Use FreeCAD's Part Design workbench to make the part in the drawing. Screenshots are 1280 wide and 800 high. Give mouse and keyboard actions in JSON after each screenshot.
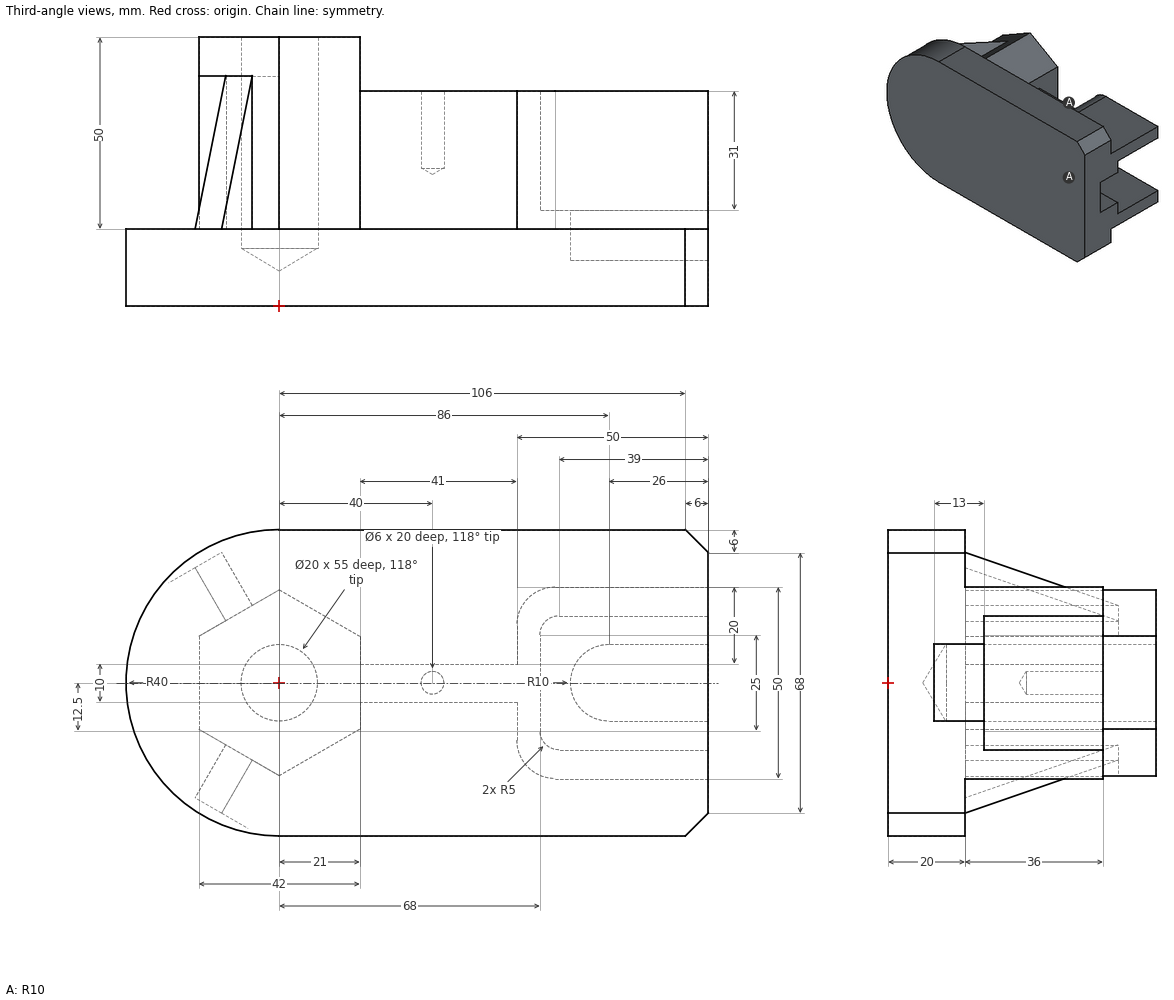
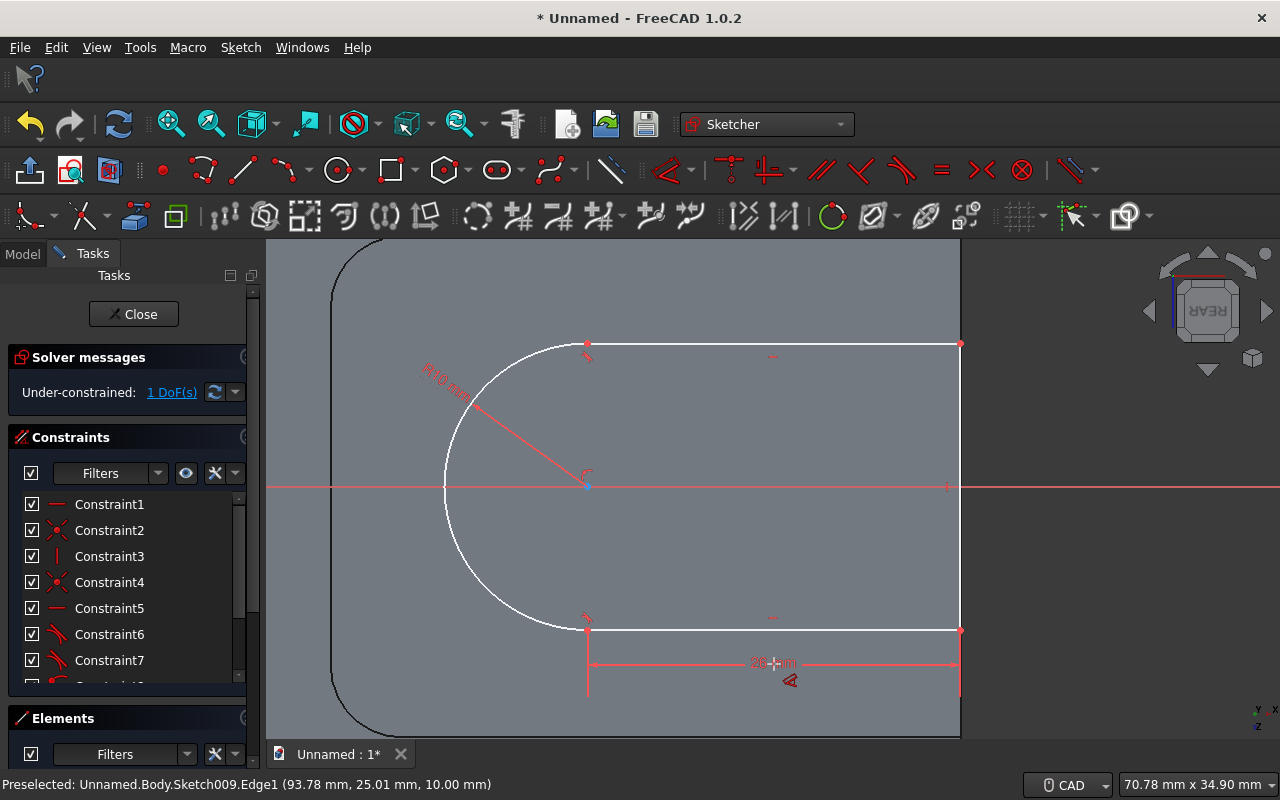
{"action": "left_click", "coordinate": [588, 630]}
{"action": "left_click", "coordinate": [441, 664]}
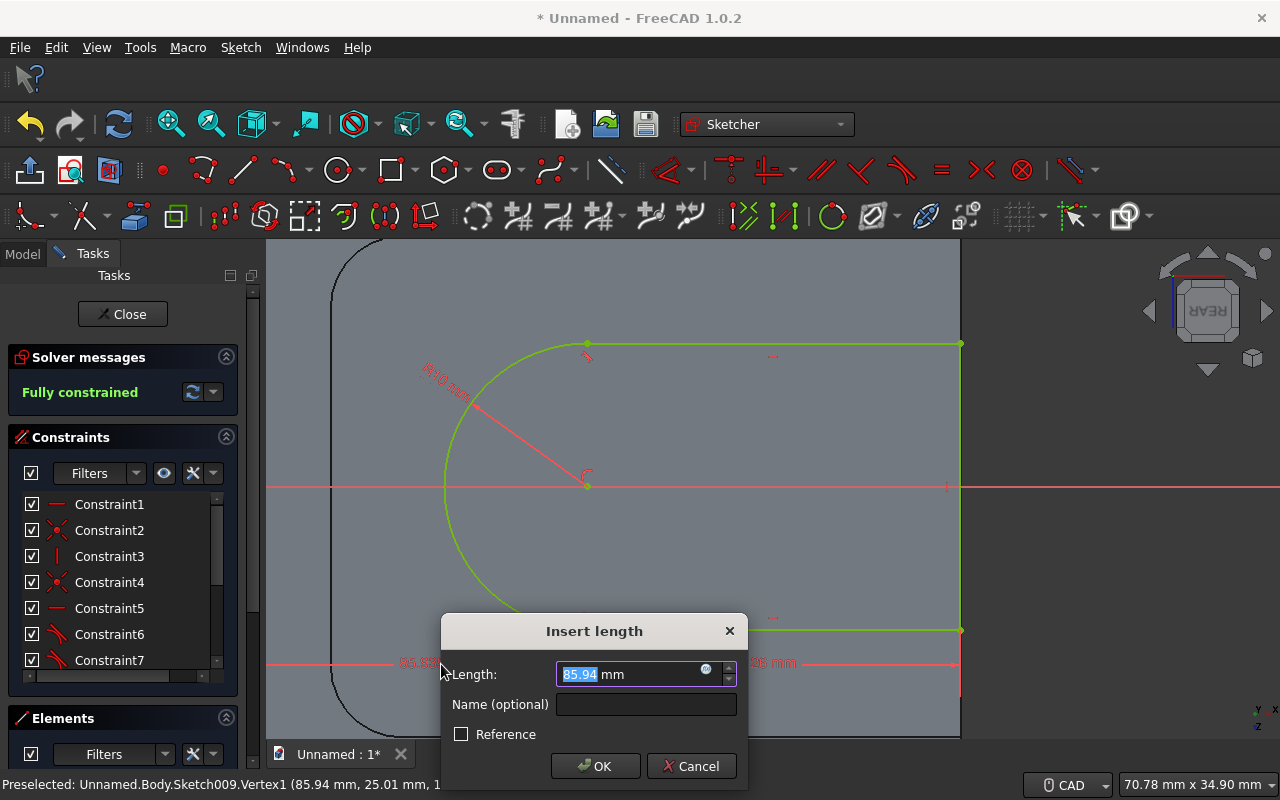
{"action": "type", "text": "86"}
{"action": "key", "text": "Return"}
{"action": "key", "text": "Escape"}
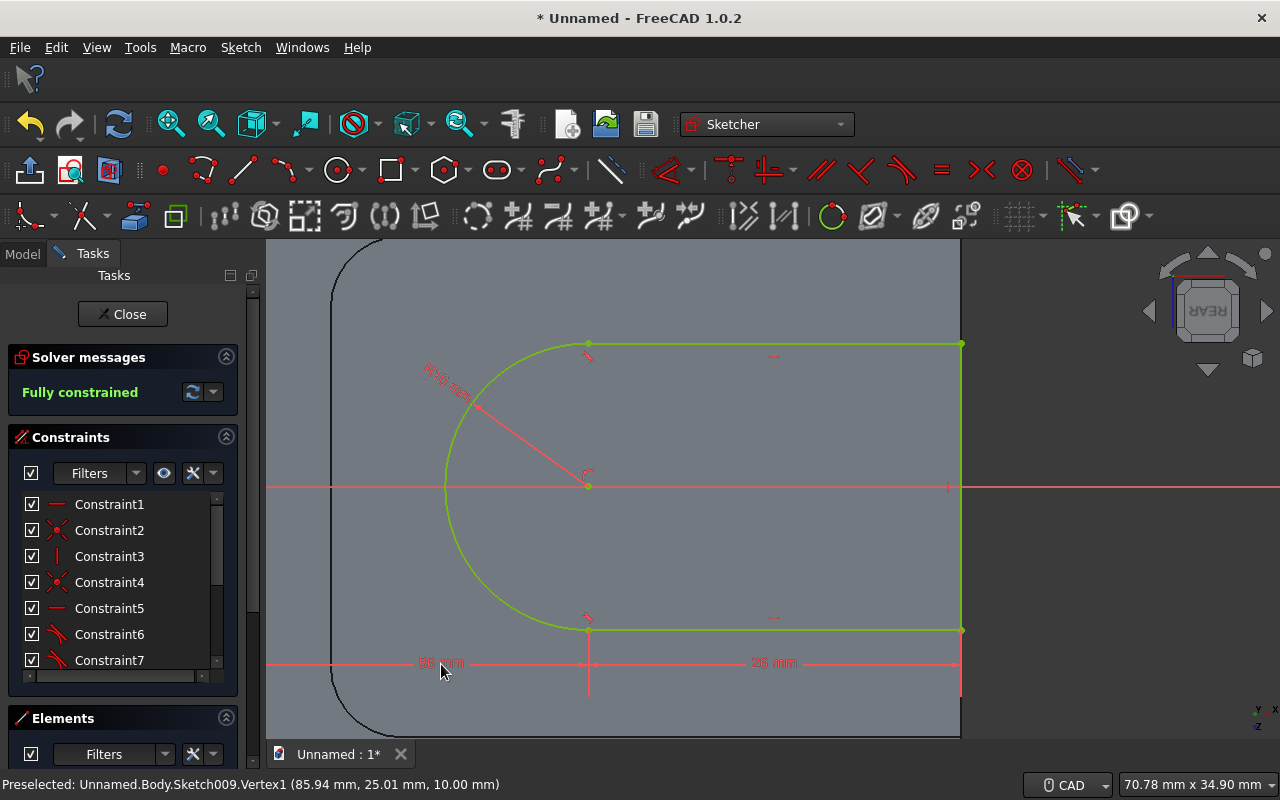
{"action": "left_click", "coordinate": [123, 314]}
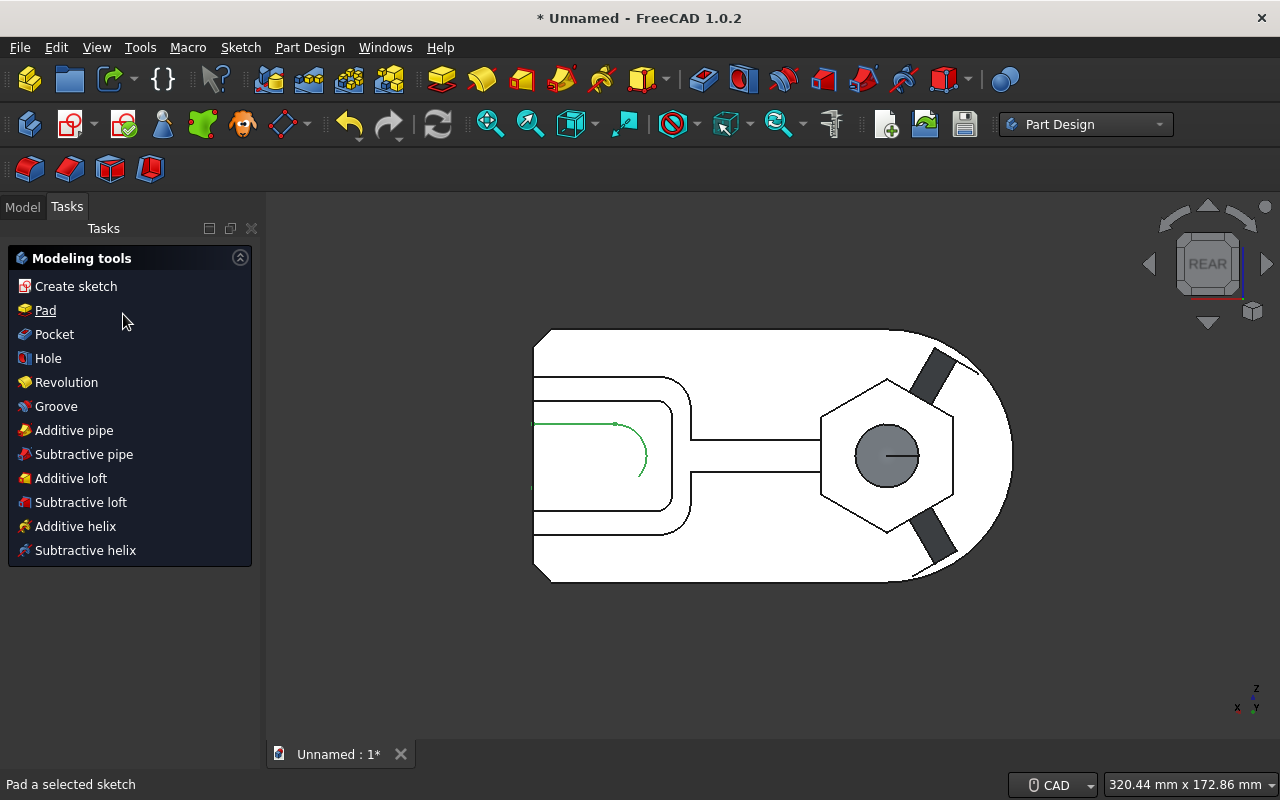
{"action": "left_click", "coordinate": [704, 80]}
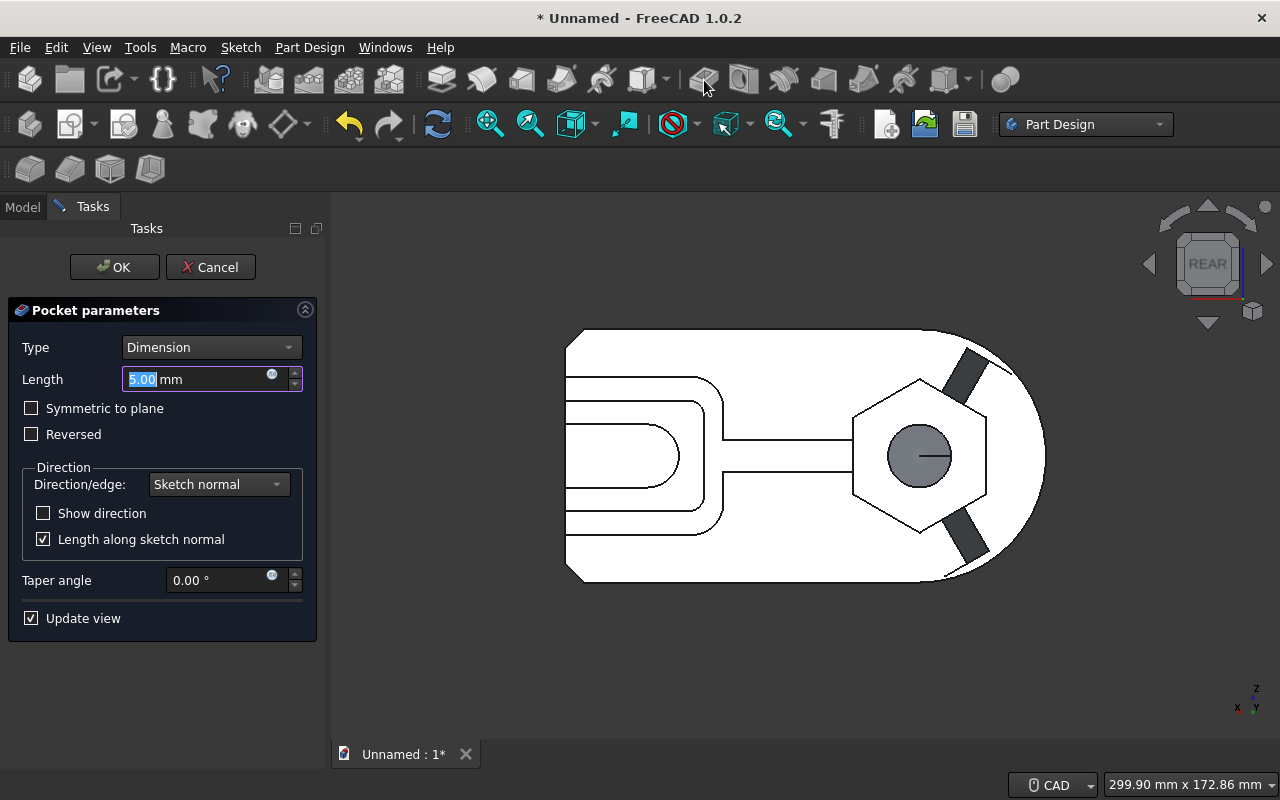
{"action": "type", "text": "13"}
{"action": "key", "text": "Tab"}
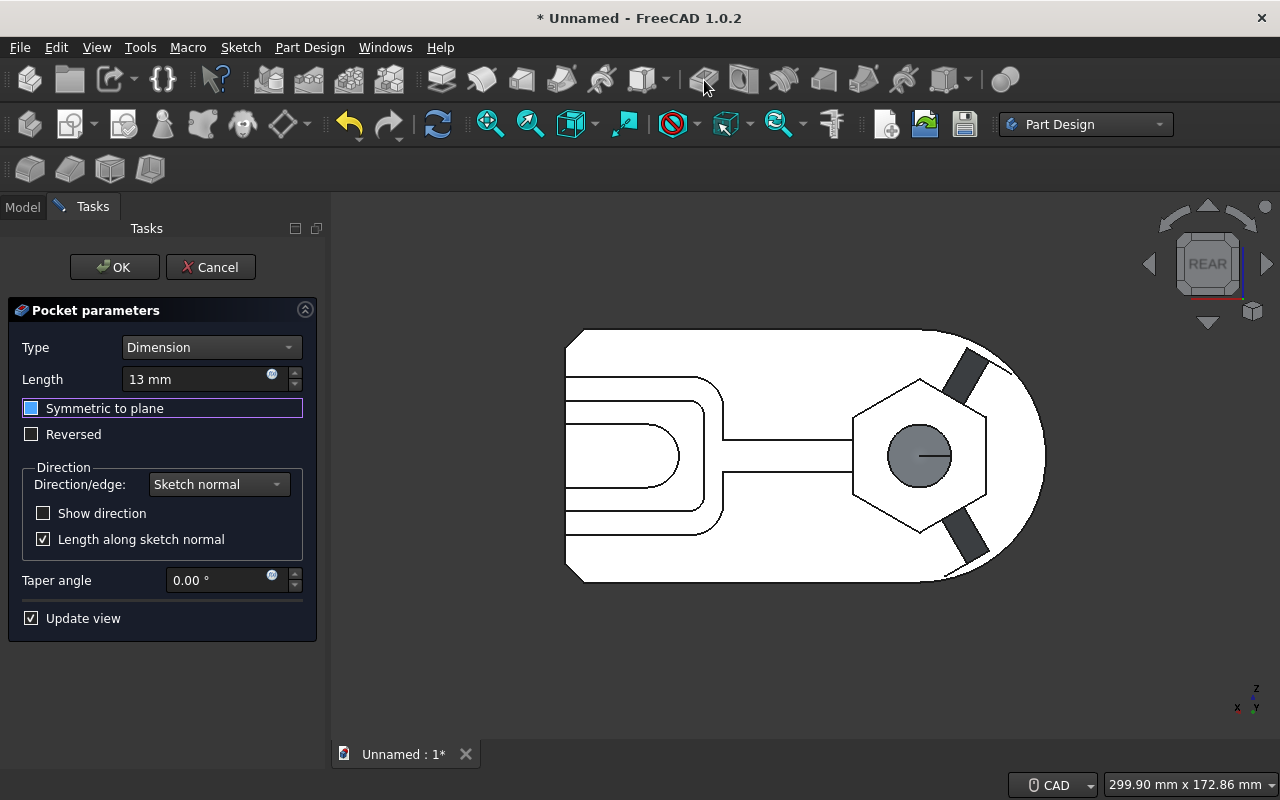
{"action": "left_click", "coordinate": [115, 267]}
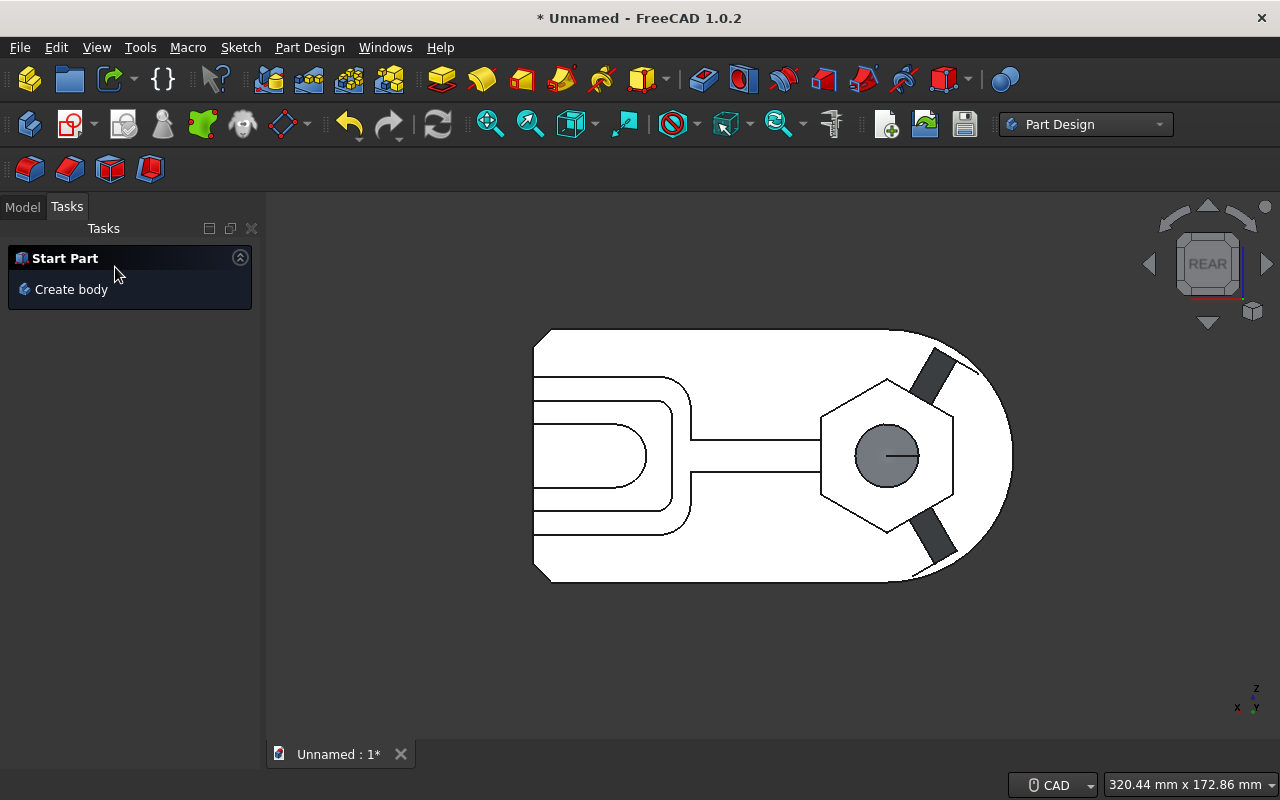
{"action": "left_click", "coordinate": [718, 455]}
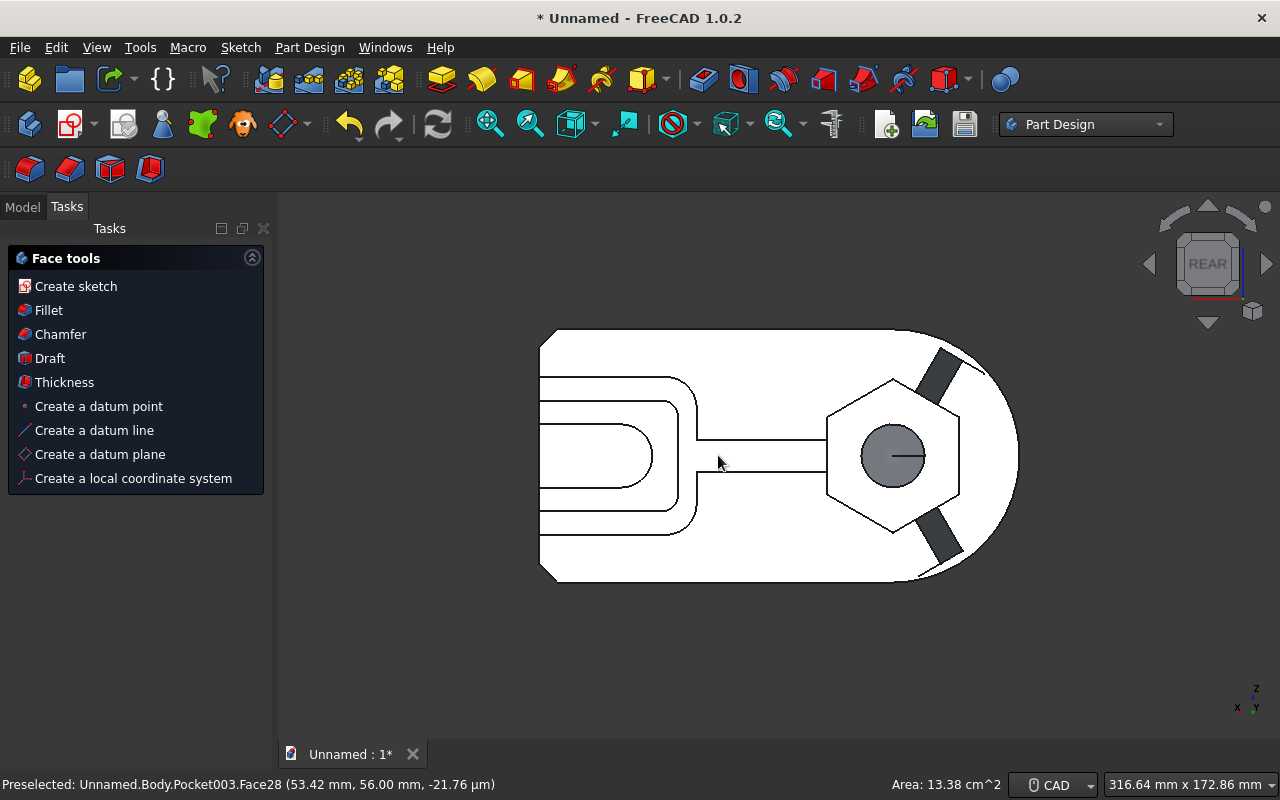
{"action": "left_click", "coordinate": [70, 124]}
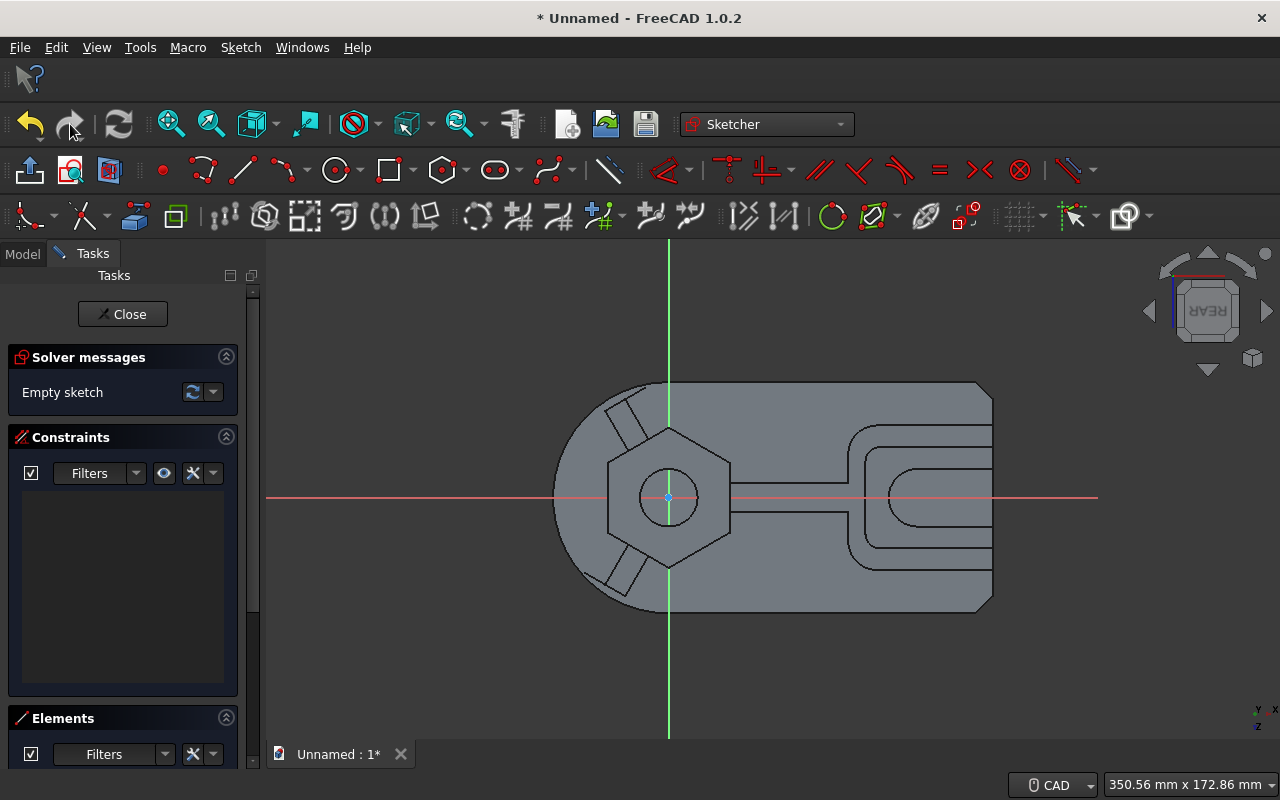
{"action": "left_click", "coordinate": [110, 170]}